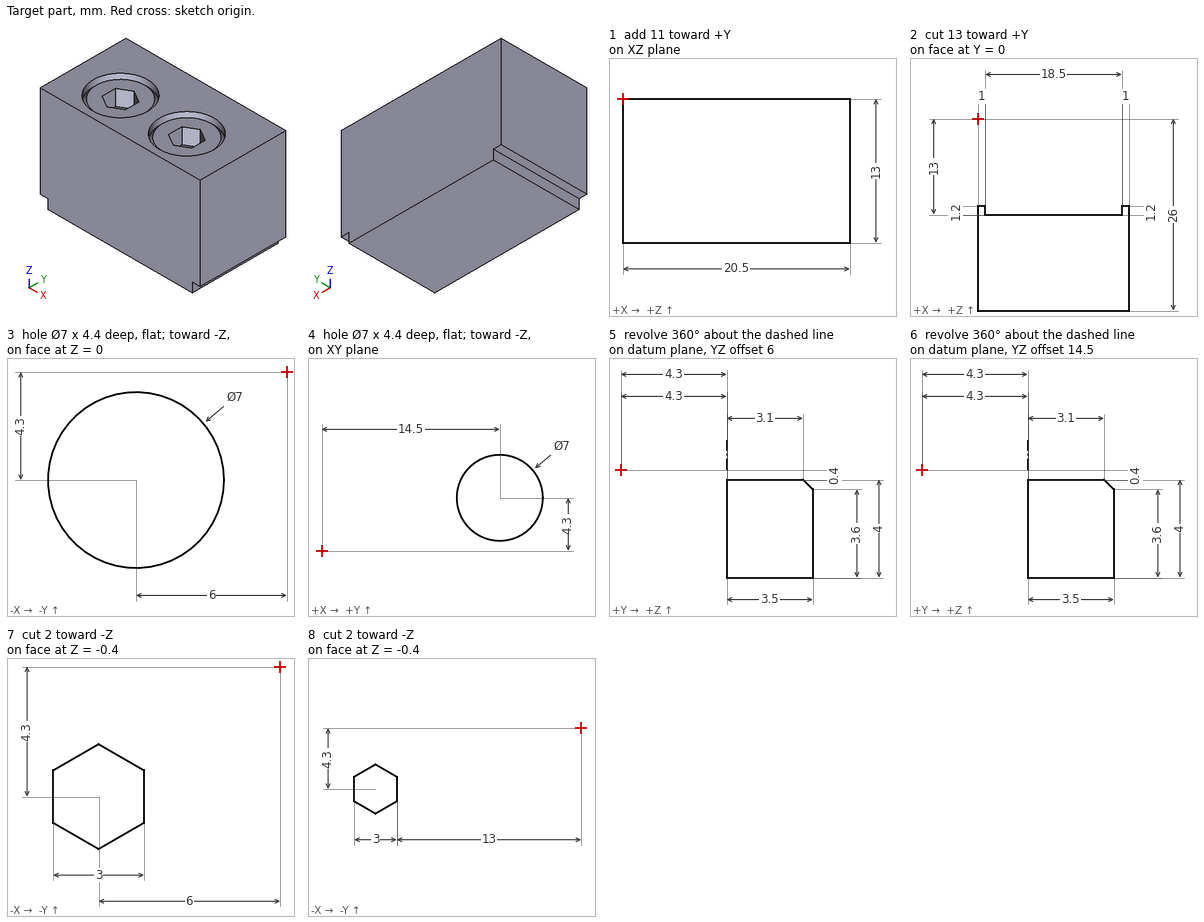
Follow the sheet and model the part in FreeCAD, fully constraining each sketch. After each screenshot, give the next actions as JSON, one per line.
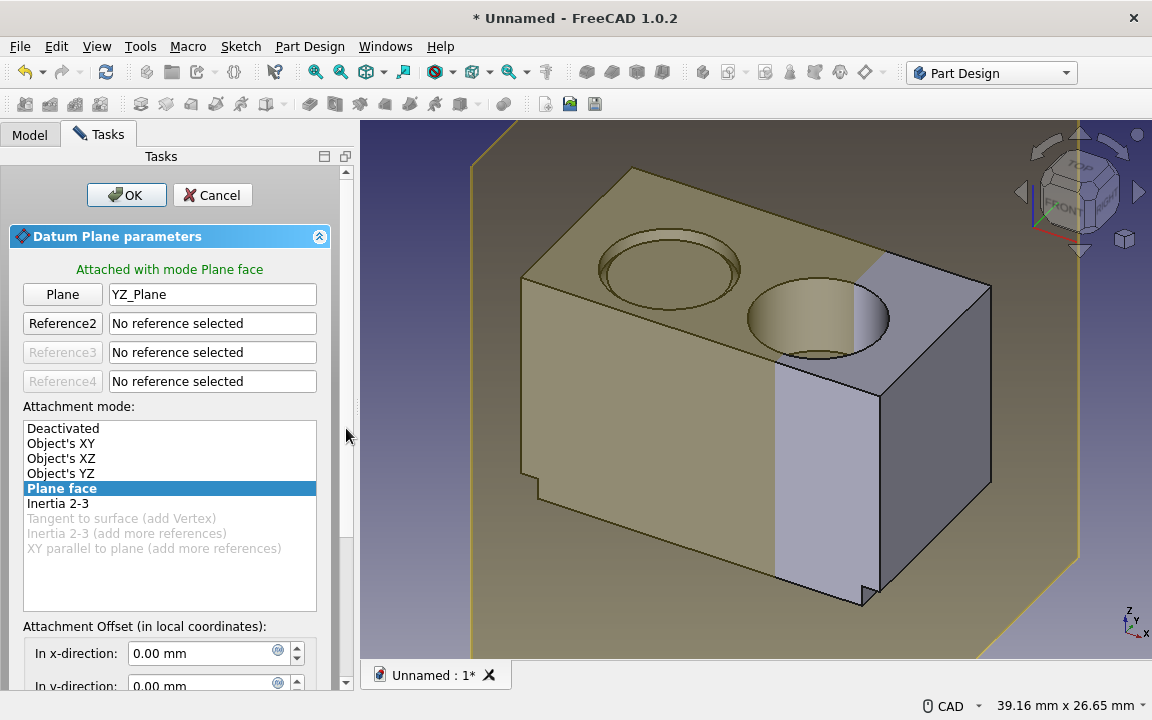
{"action": "left_click", "coordinate": [127, 195]}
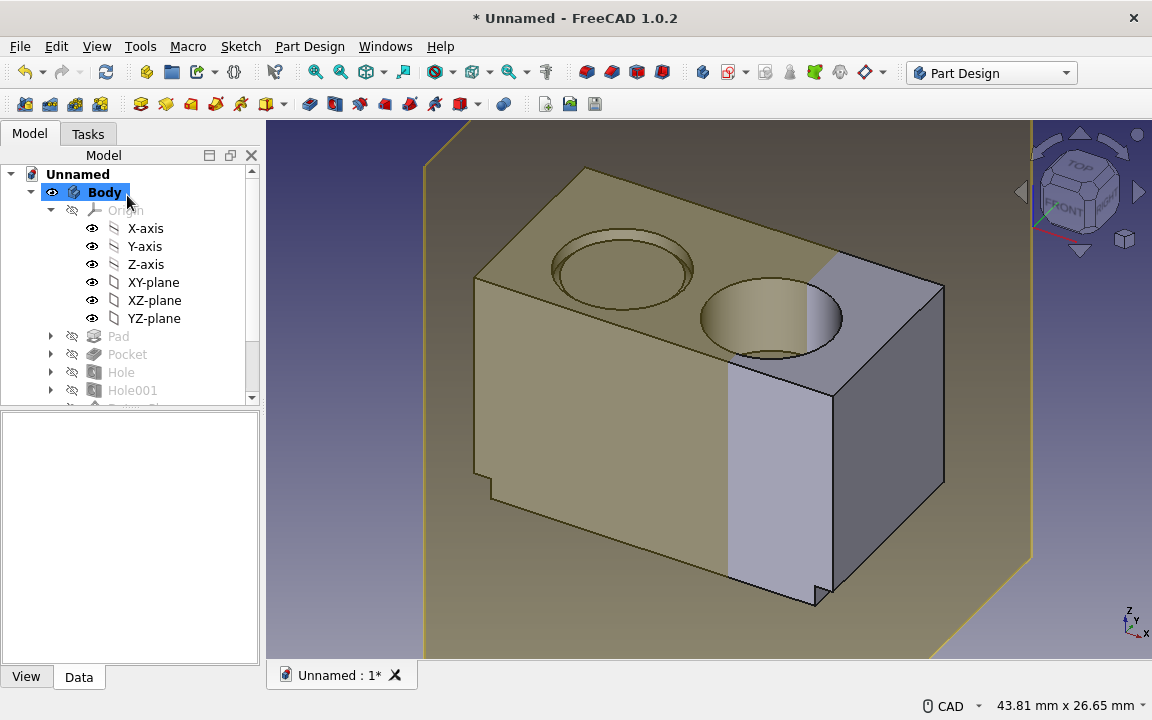
{"action": "scroll", "coordinate": [101, 278], "scroll_direction": "down", "scroll_amount": 3}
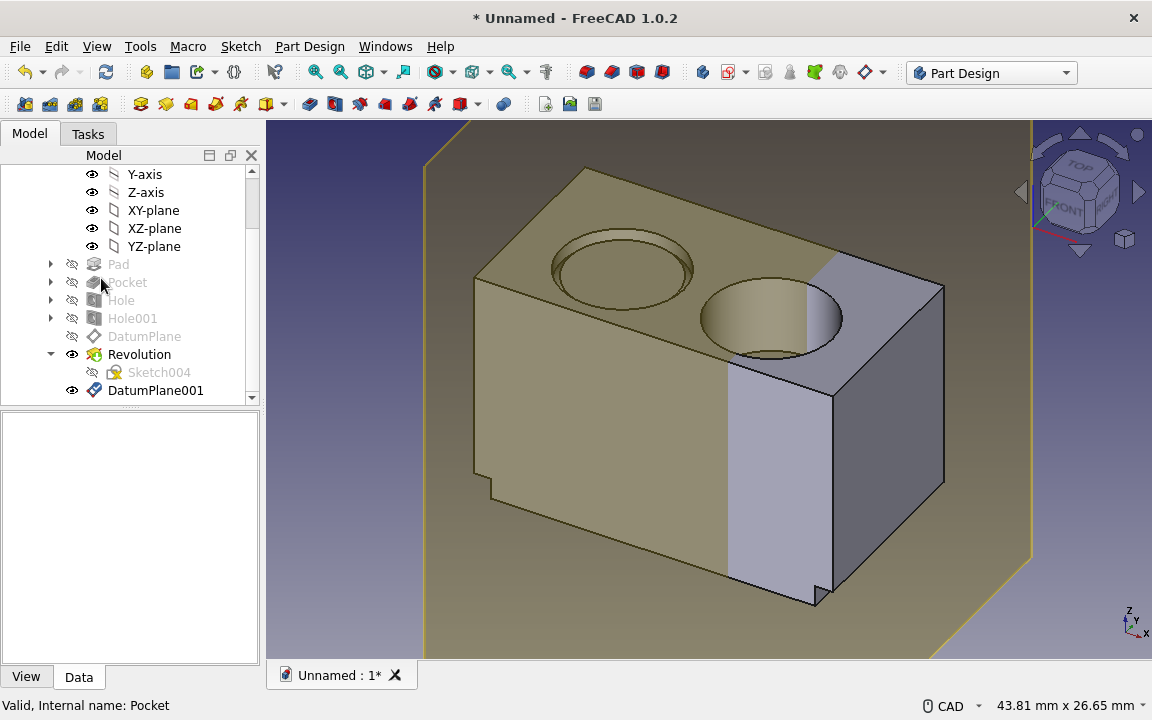
{"action": "left_click", "coordinate": [117, 390]}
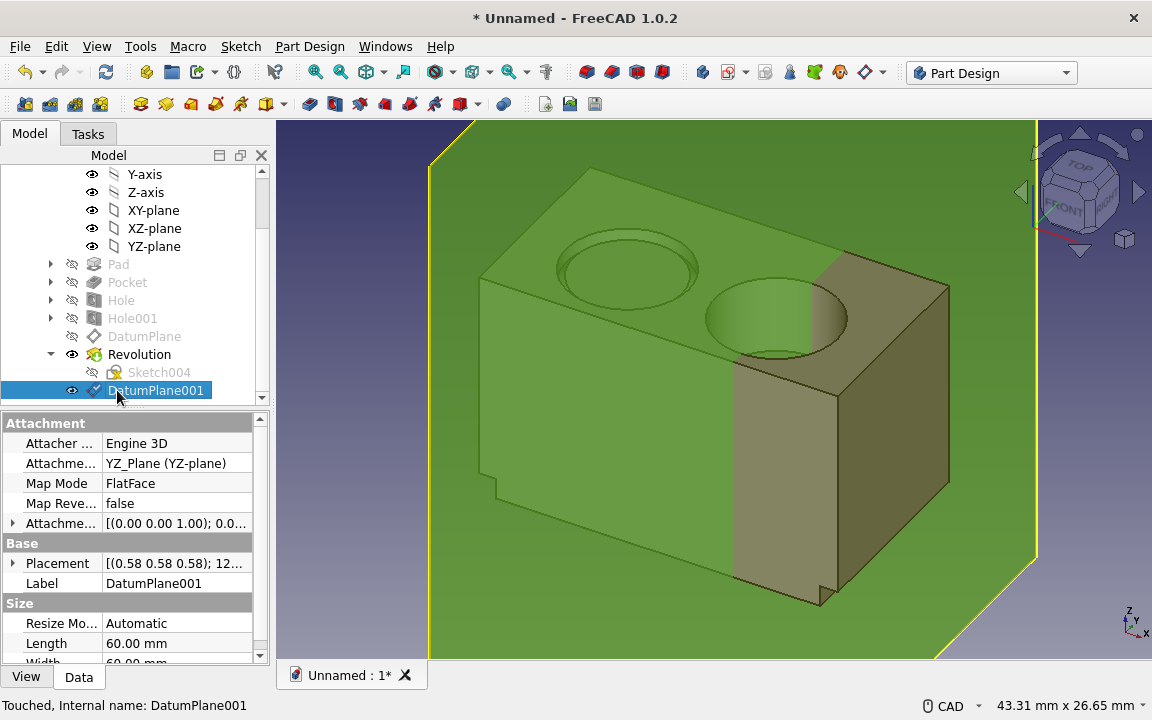
{"action": "left_click", "coordinate": [728, 72]}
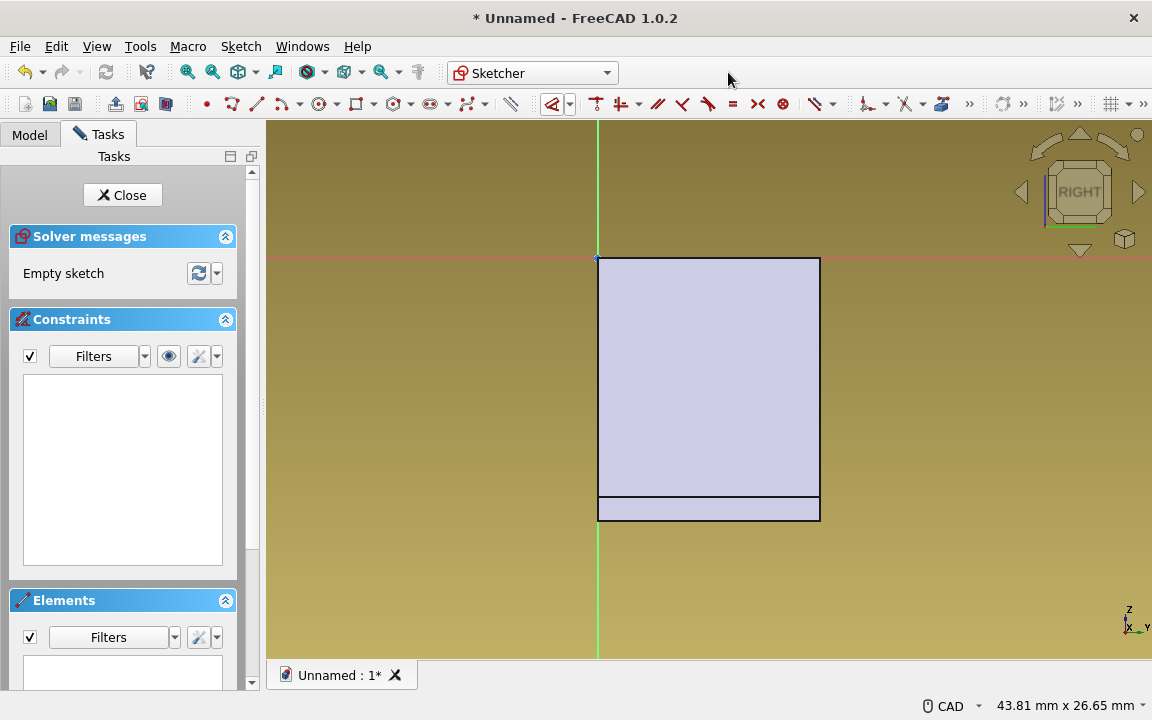
{"action": "left_click", "coordinate": [166, 104]}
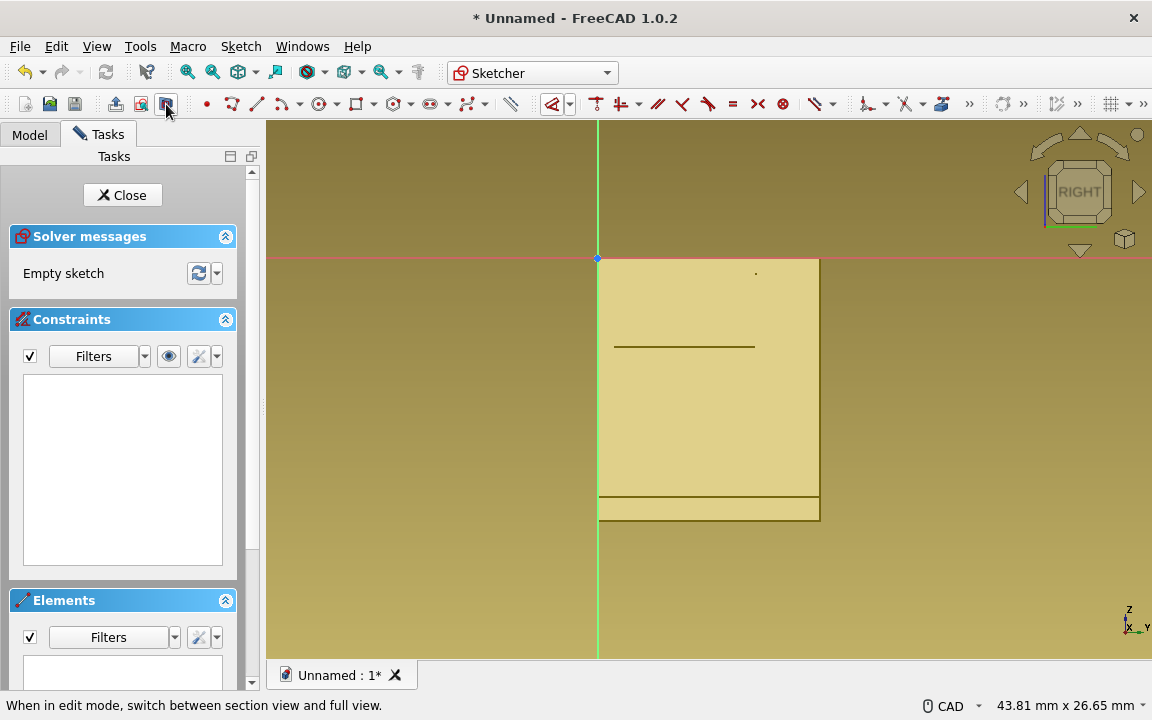
{"action": "scroll", "coordinate": [692, 248], "scroll_direction": "up", "scroll_amount": 6}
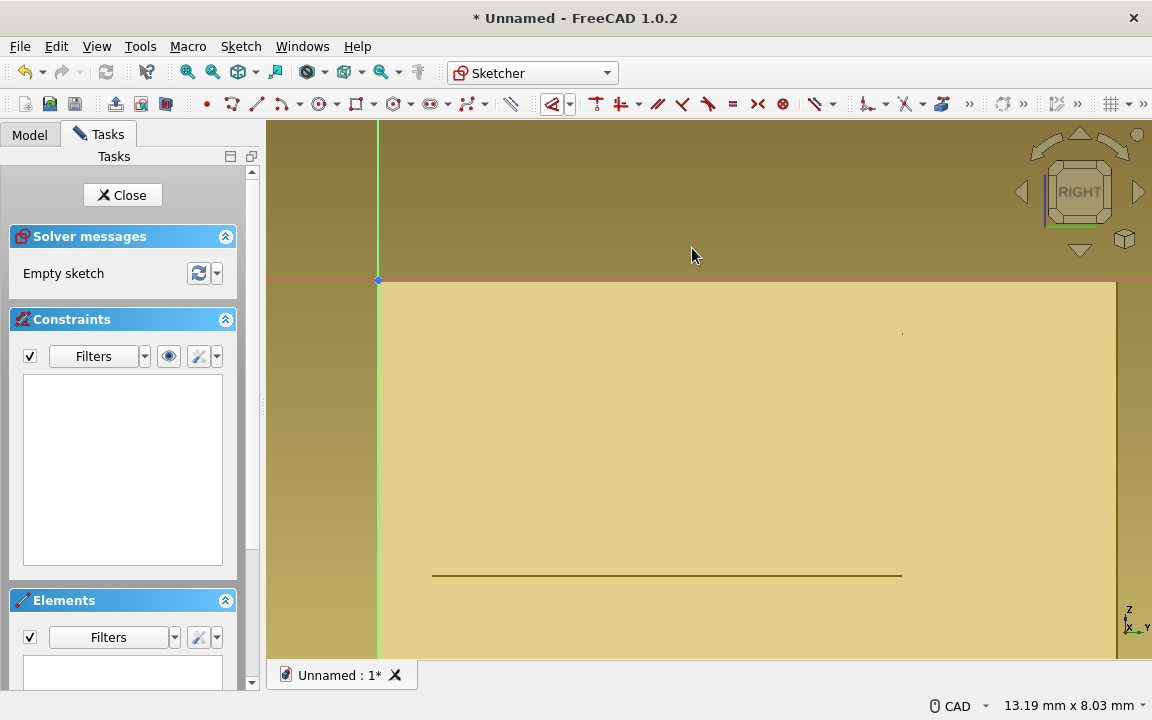
{"action": "left_click", "coordinate": [232, 104]}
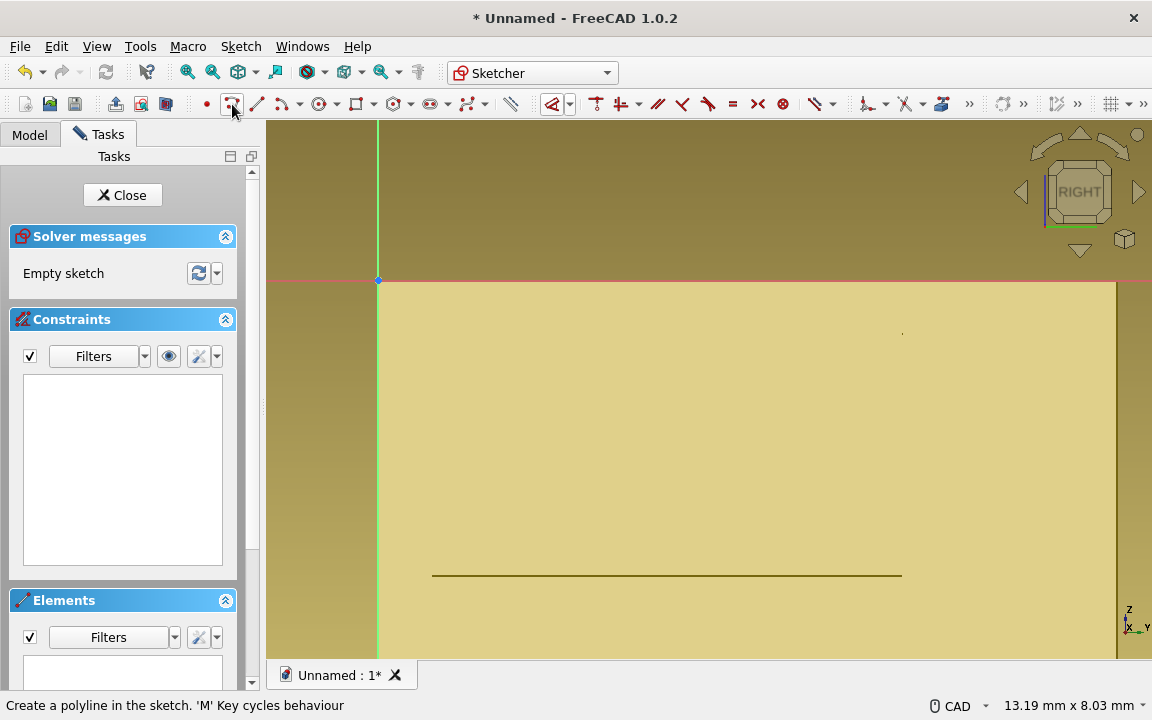
{"action": "left_click", "coordinate": [667, 308]}
{"action": "left_click", "coordinate": [667, 576]}
{"action": "left_click", "coordinate": [902, 576]}
{"action": "left_click", "coordinate": [902, 334]}
{"action": "left_click", "coordinate": [875, 308]}
{"action": "left_click", "coordinate": [667, 309]}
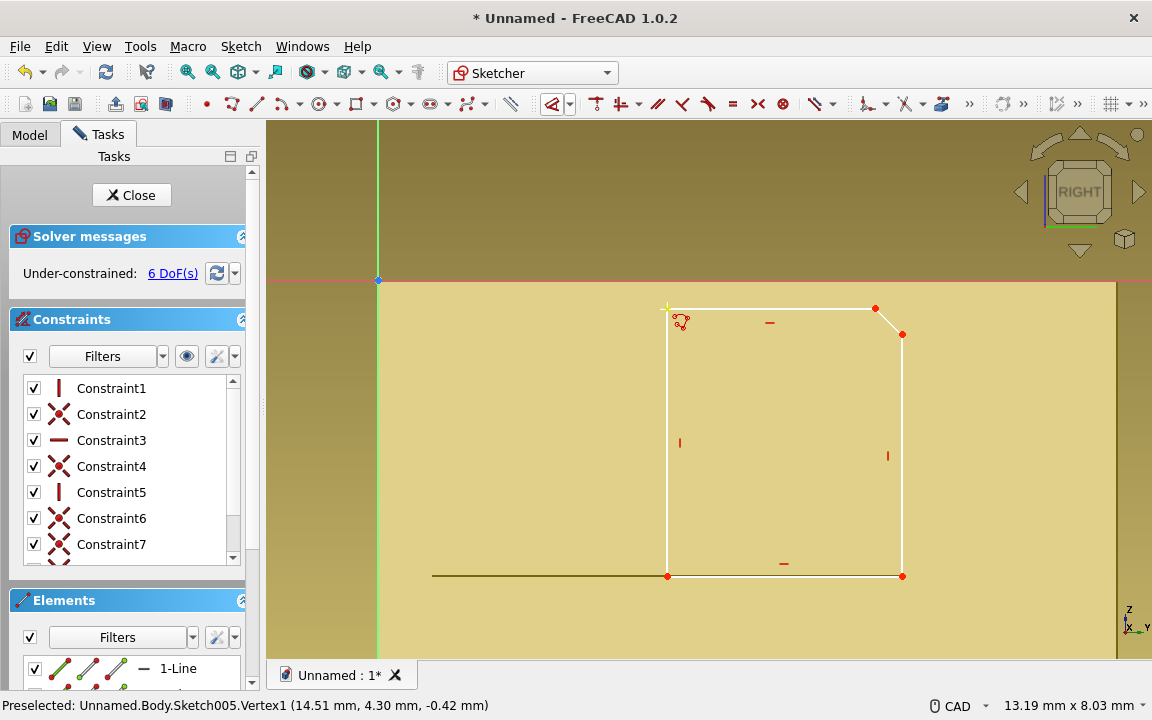
{"action": "key", "text": "g l"}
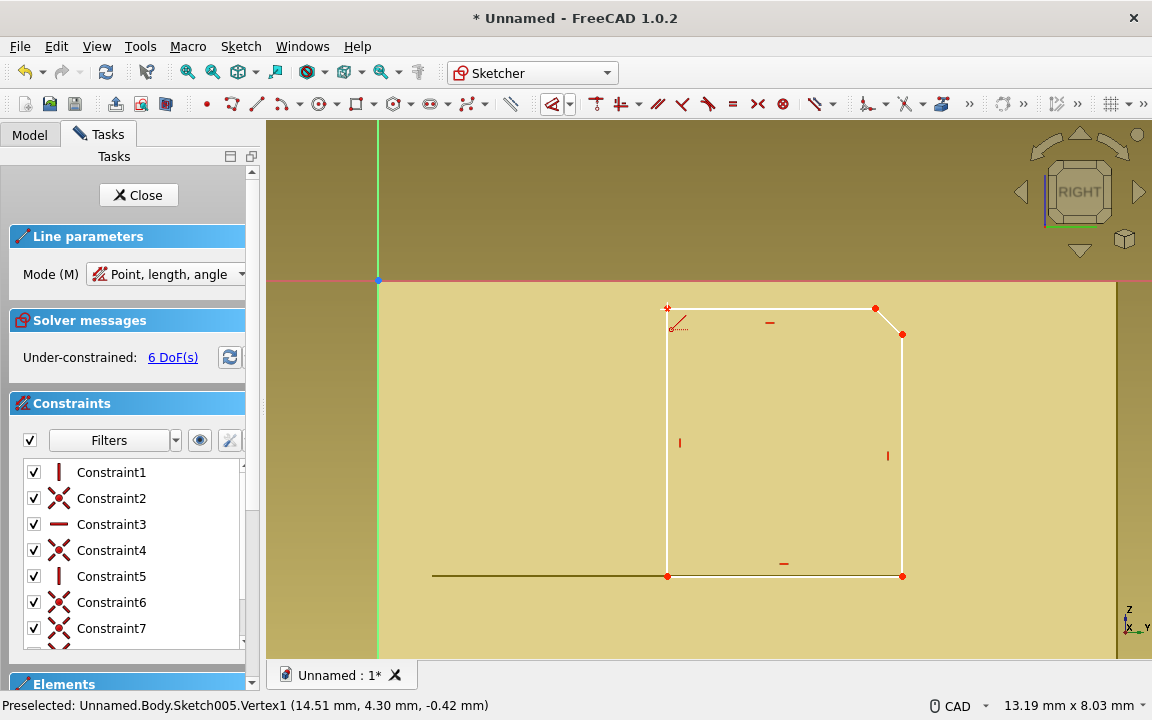
{"action": "left_click", "coordinate": [667, 281]}
{"action": "left_click", "coordinate": [667, 200]}
{"action": "key", "text": "Escape"}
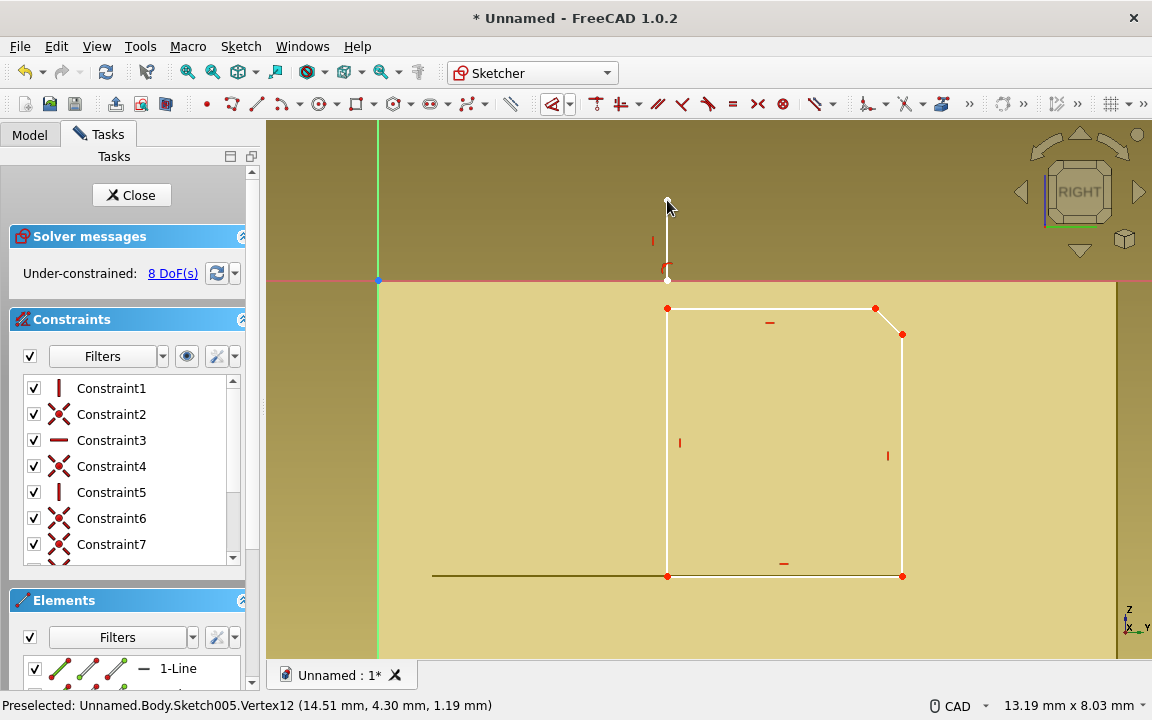
{"action": "left_click", "coordinate": [667, 257]}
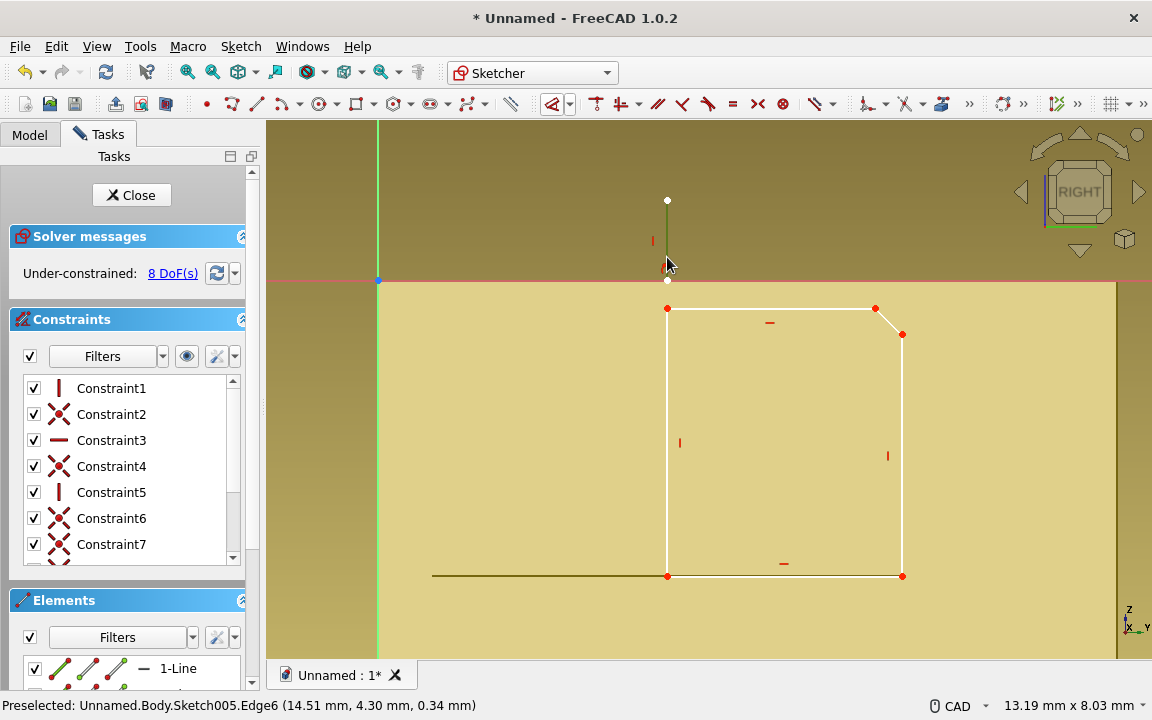
{"action": "left_click", "coordinate": [511, 104]}